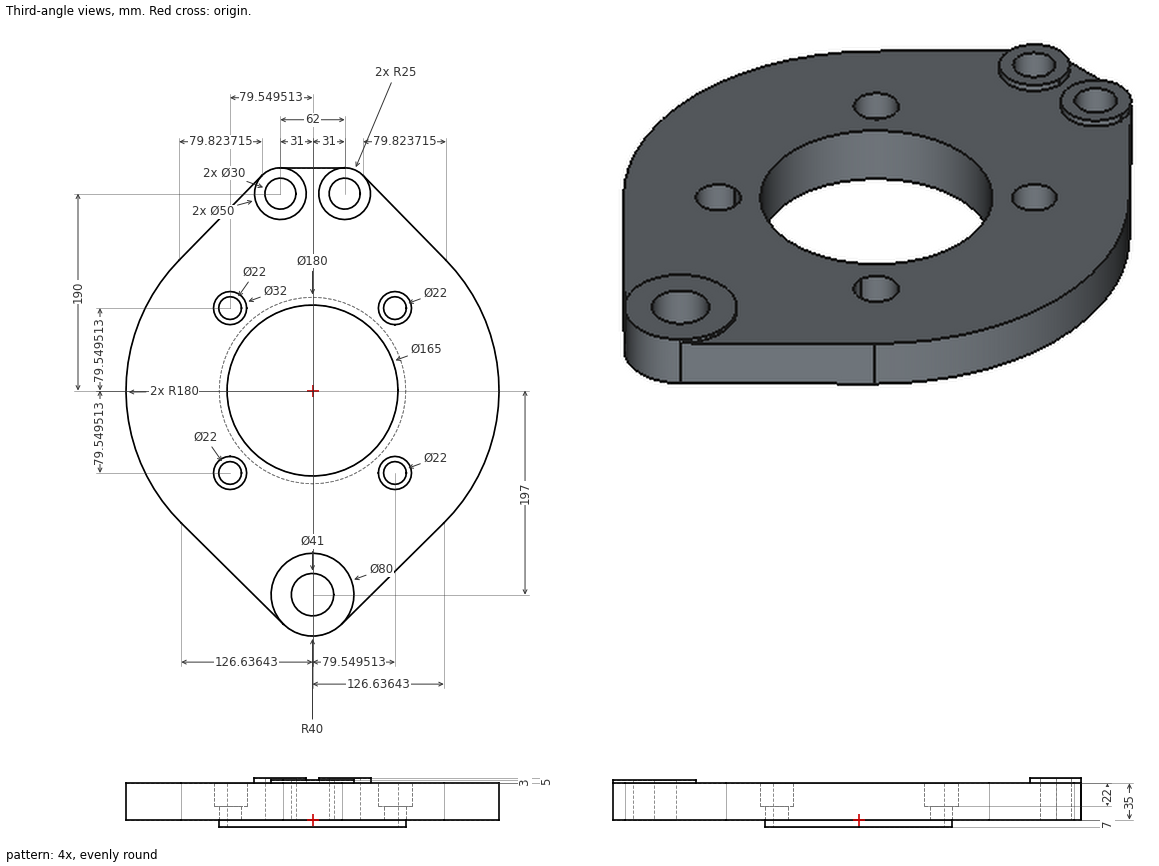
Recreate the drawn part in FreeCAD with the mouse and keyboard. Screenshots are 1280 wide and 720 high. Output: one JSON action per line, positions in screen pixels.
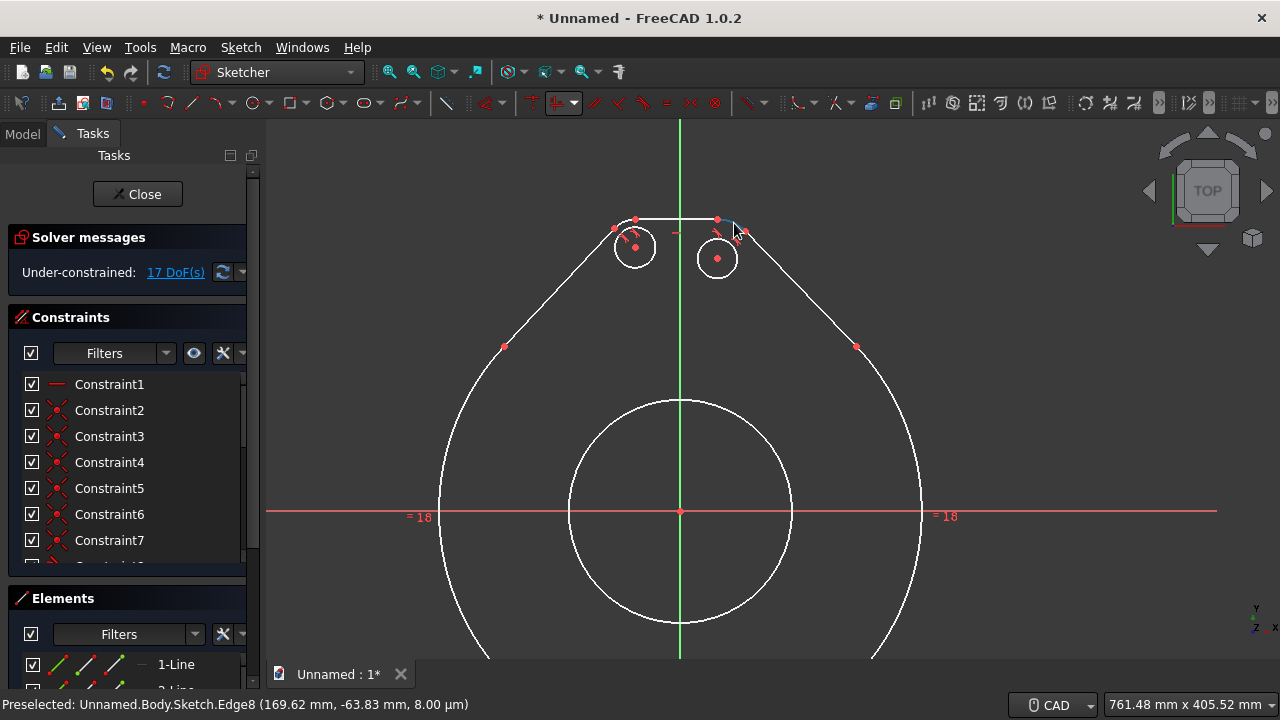
{"action": "left_click", "coordinate": [733, 223]}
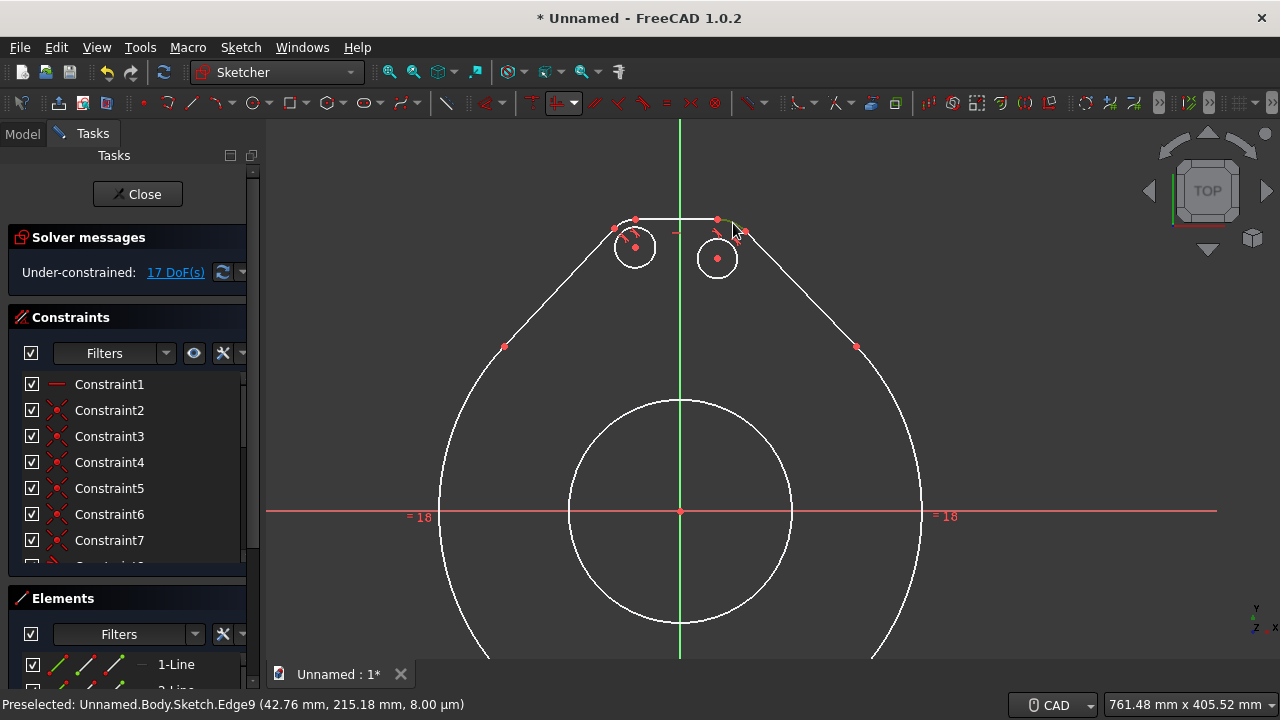
{"action": "scroll", "coordinate": [624, 222], "scroll_direction": "up", "scroll_amount": 3}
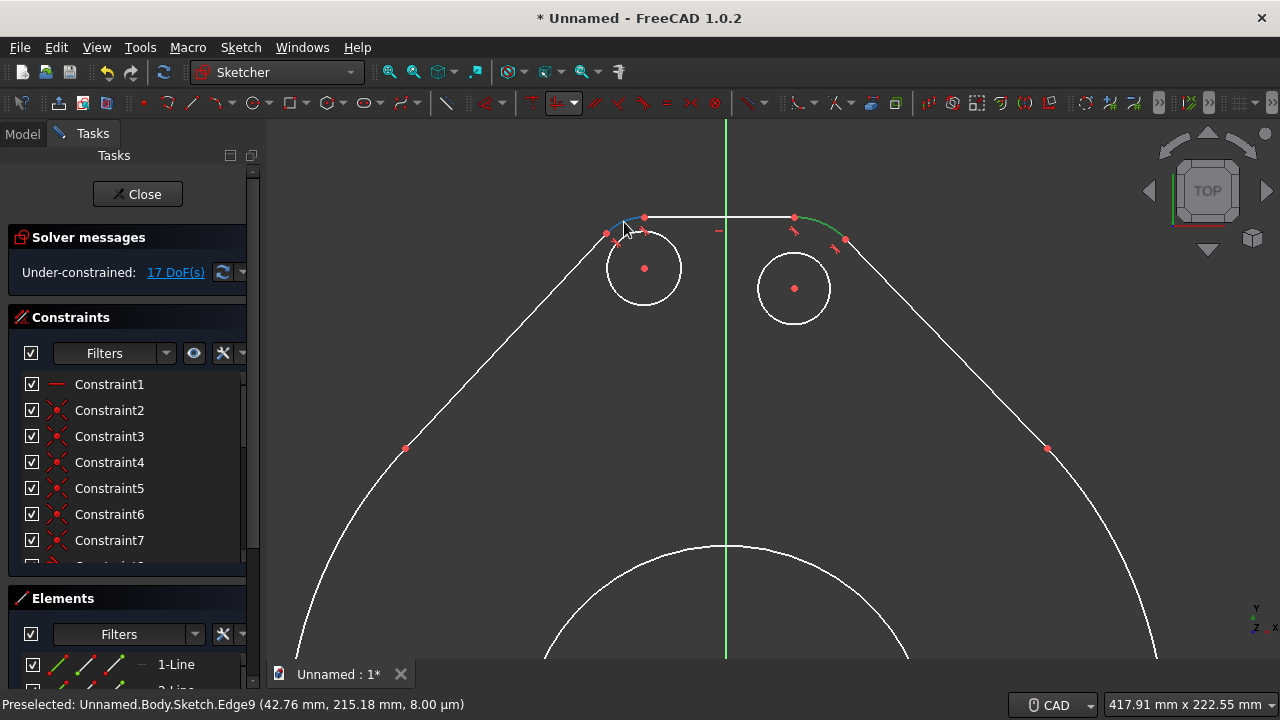
{"action": "left_click", "coordinate": [624, 221]}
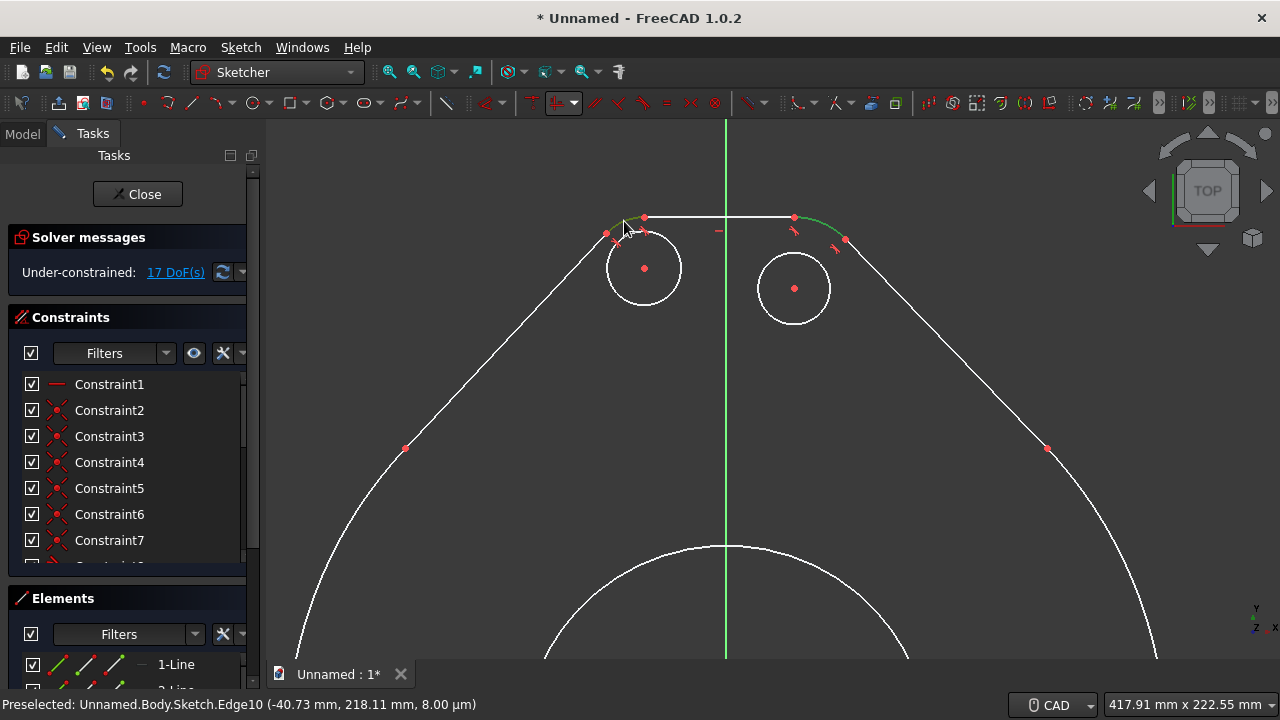
{"action": "key", "text": "e"}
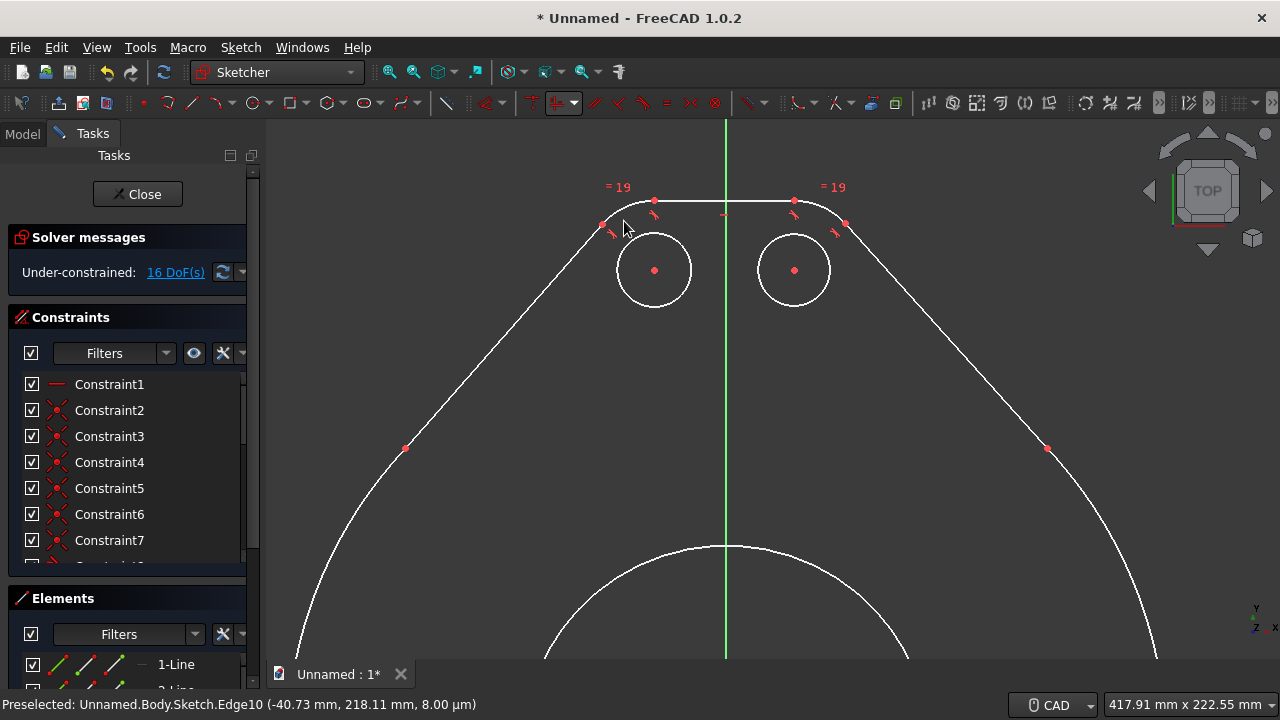
{"action": "left_click", "coordinate": [680, 244]}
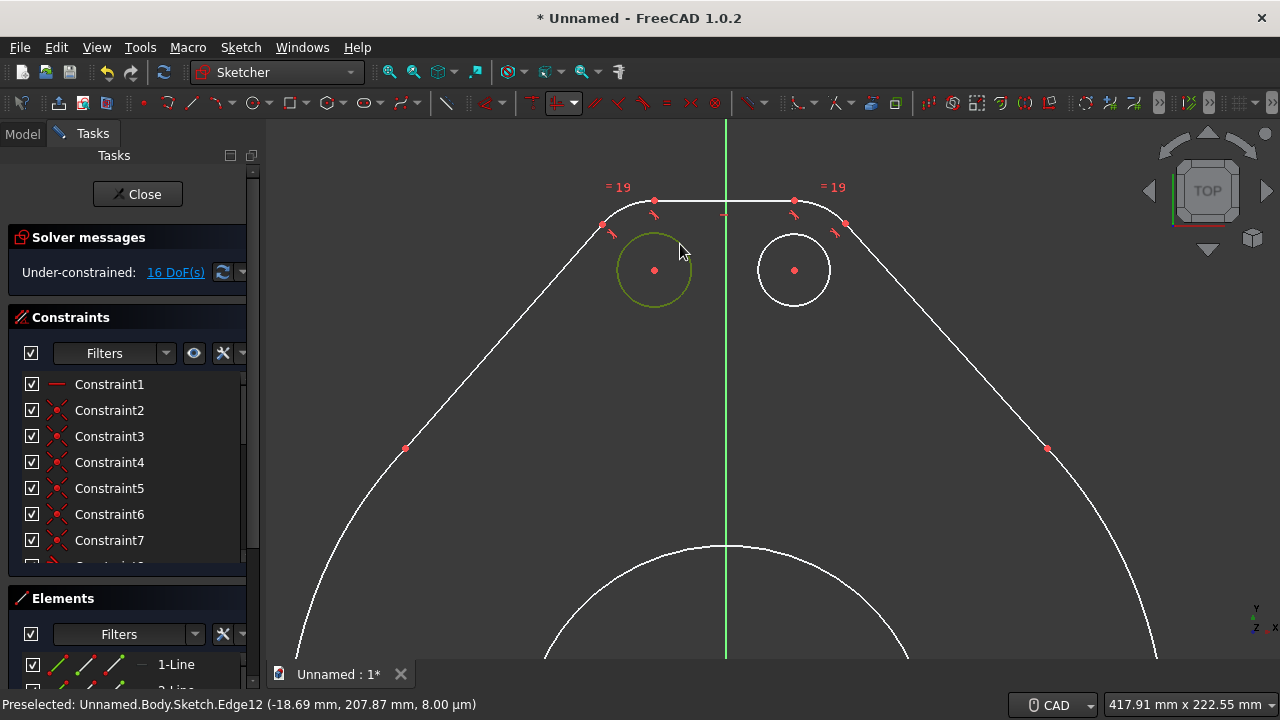
{"action": "left_click", "coordinate": [819, 245]}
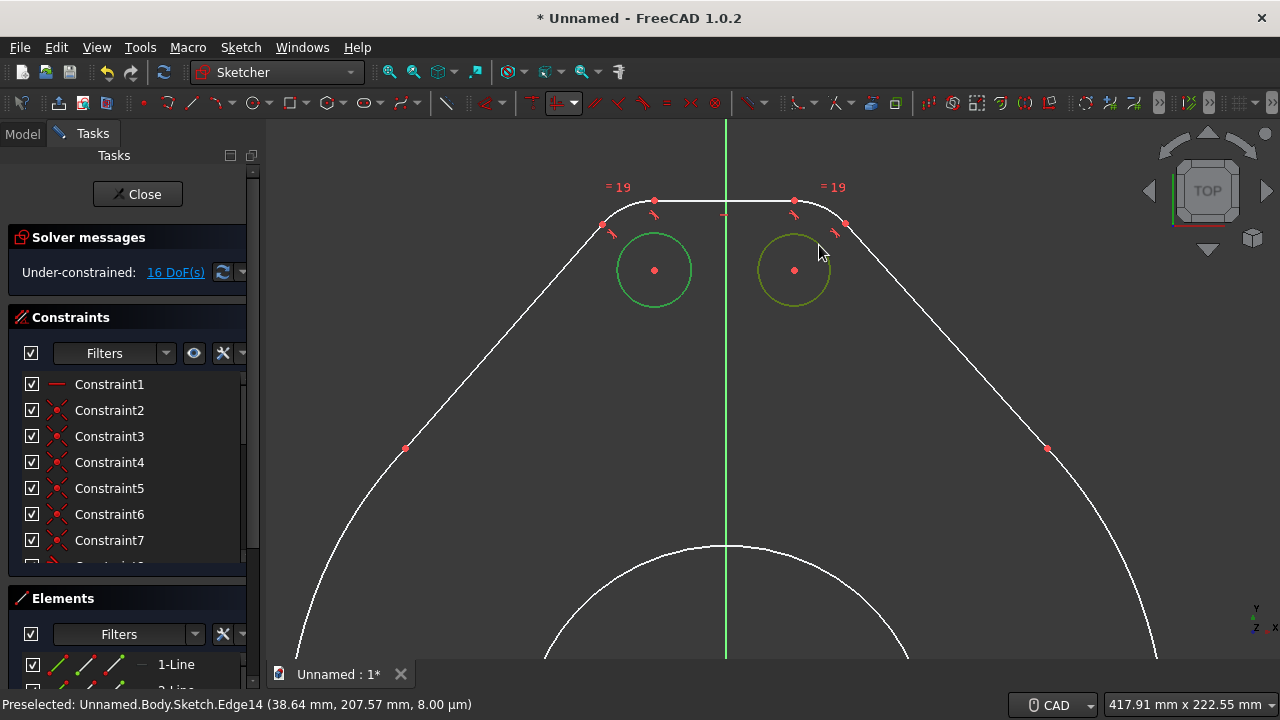
{"action": "key", "text": "e"}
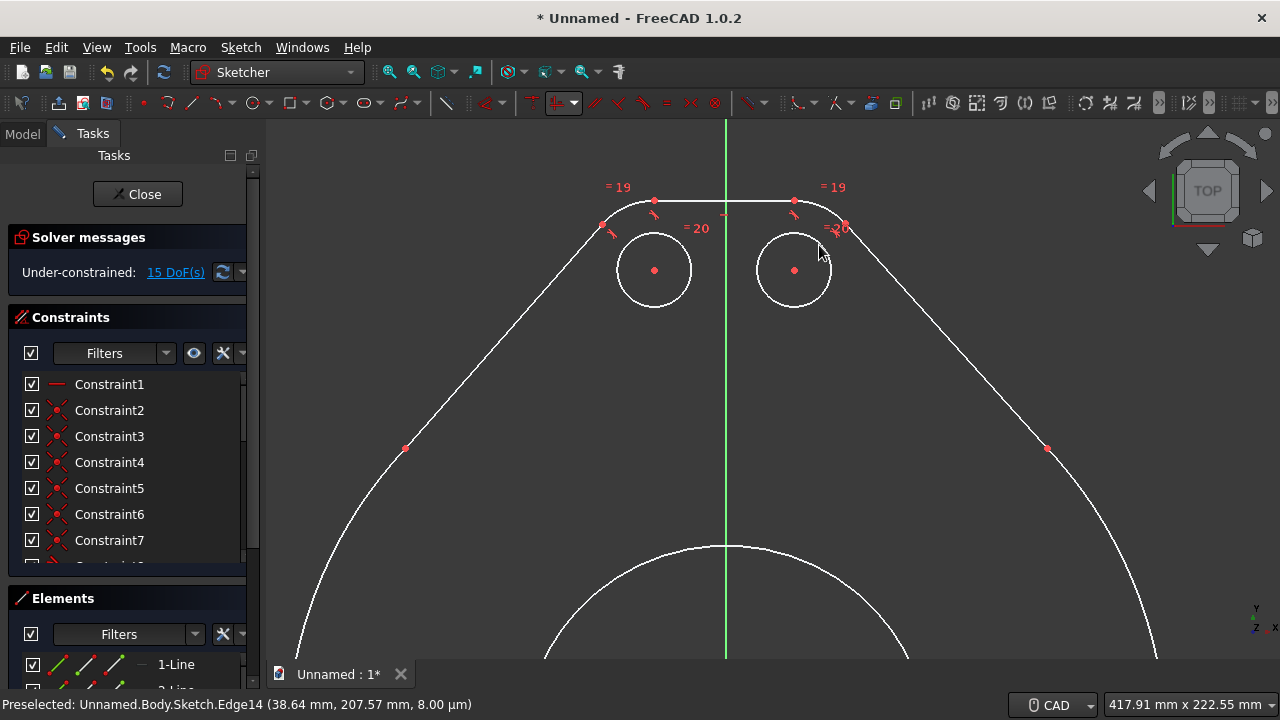
{"action": "scroll", "coordinate": [695, 222], "scroll_direction": "down", "scroll_amount": 6}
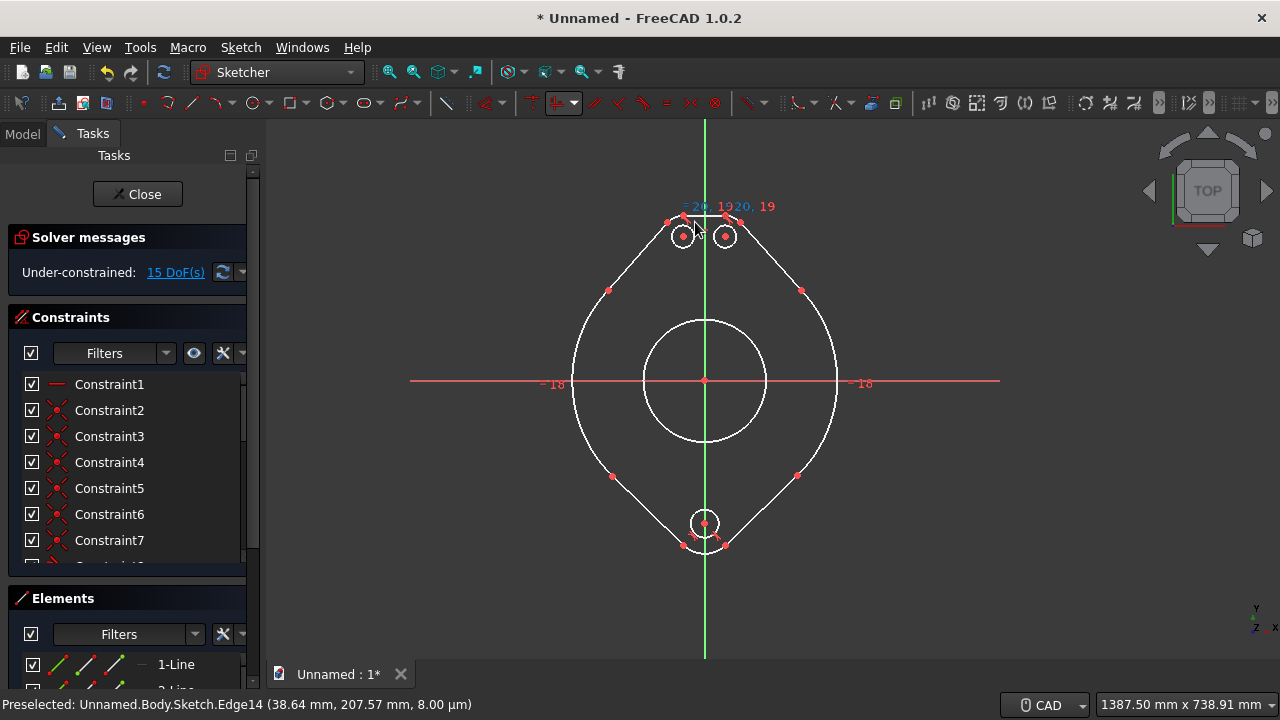
{"action": "left_click", "coordinate": [705, 524]}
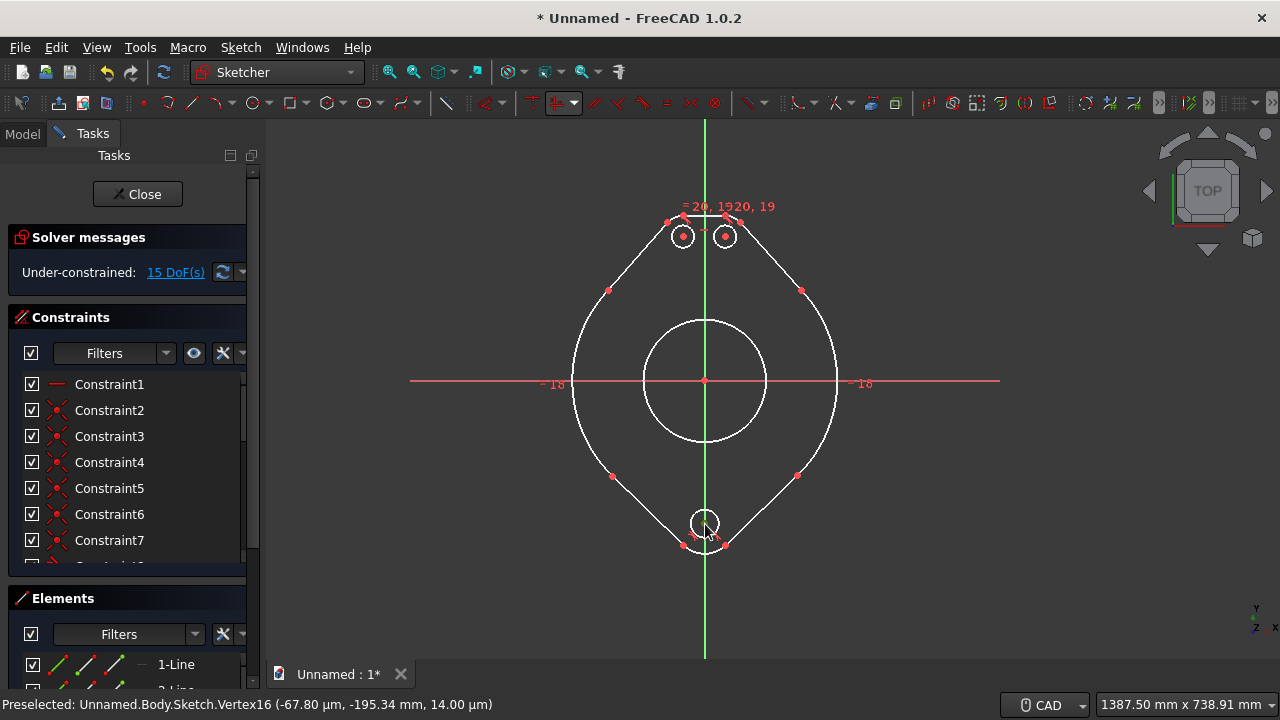
{"action": "left_click", "coordinate": [705, 596]}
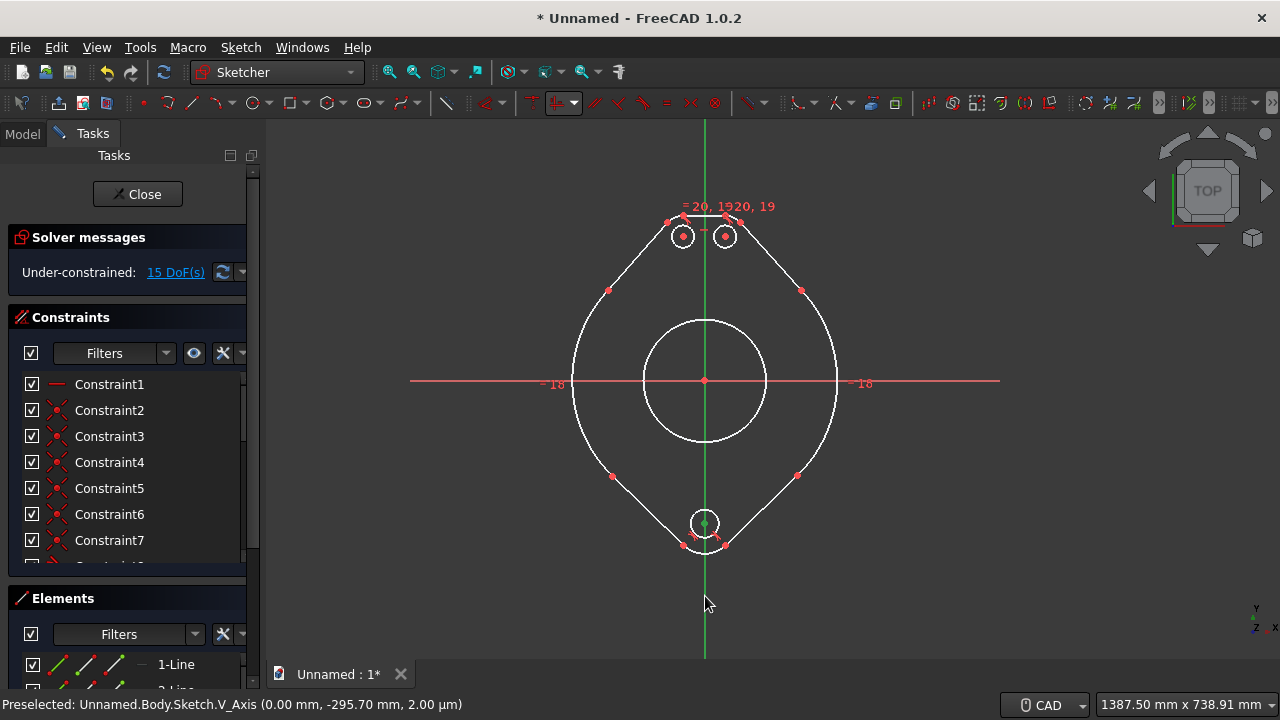
{"action": "key", "text": "c"}